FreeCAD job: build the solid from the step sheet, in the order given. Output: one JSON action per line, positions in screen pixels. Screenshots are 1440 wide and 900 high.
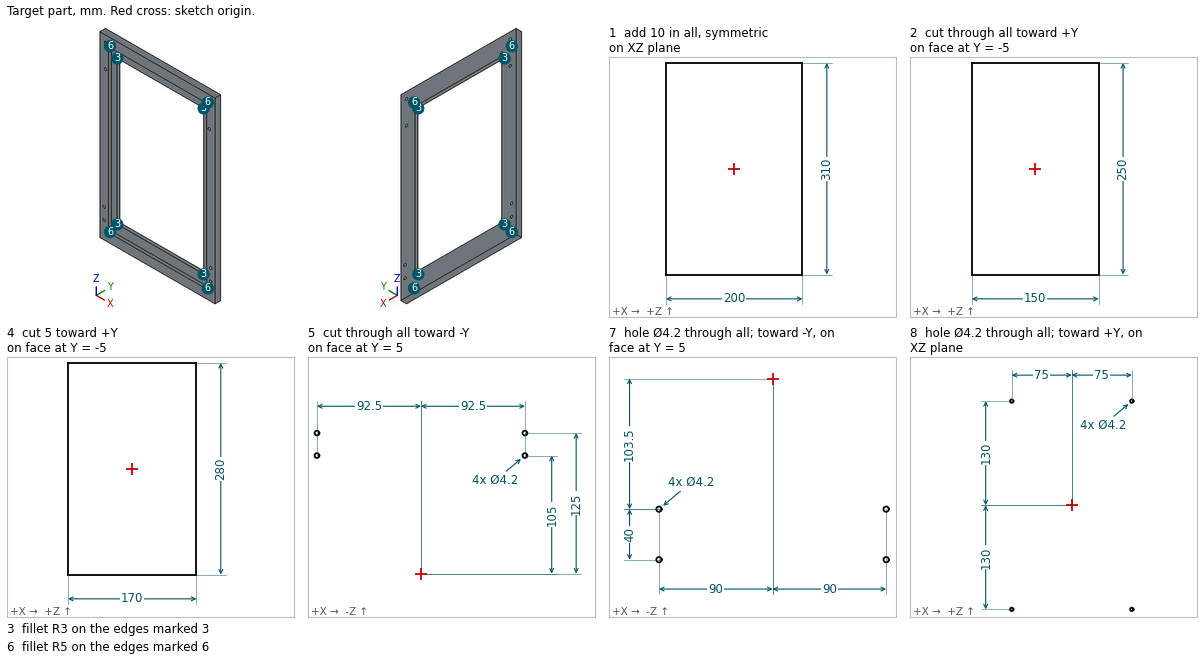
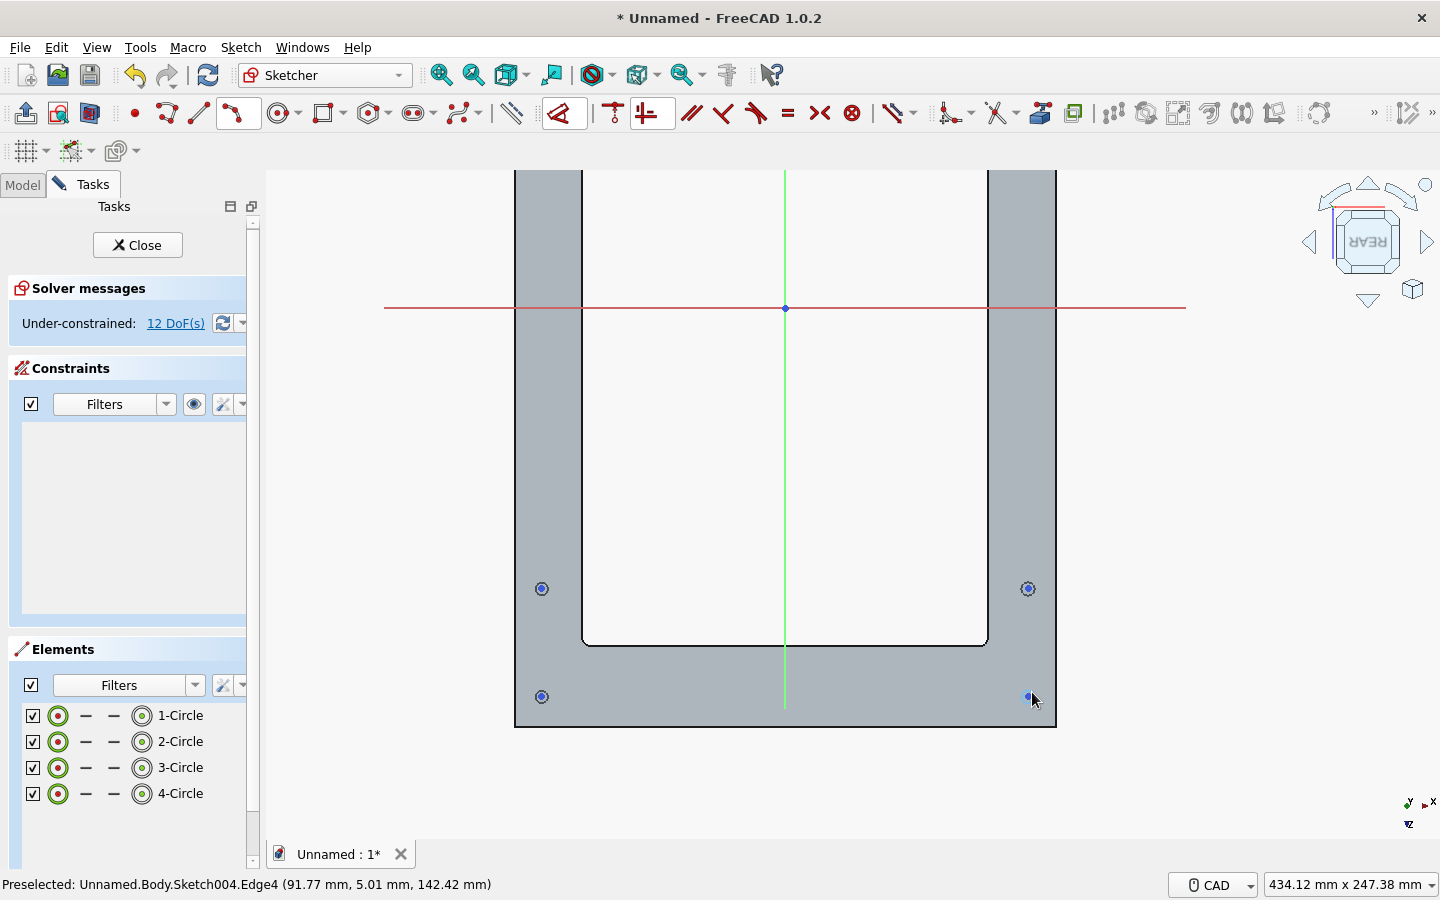
{"action": "scroll", "coordinate": [546, 585], "scroll_direction": "up", "scroll_amount": 4}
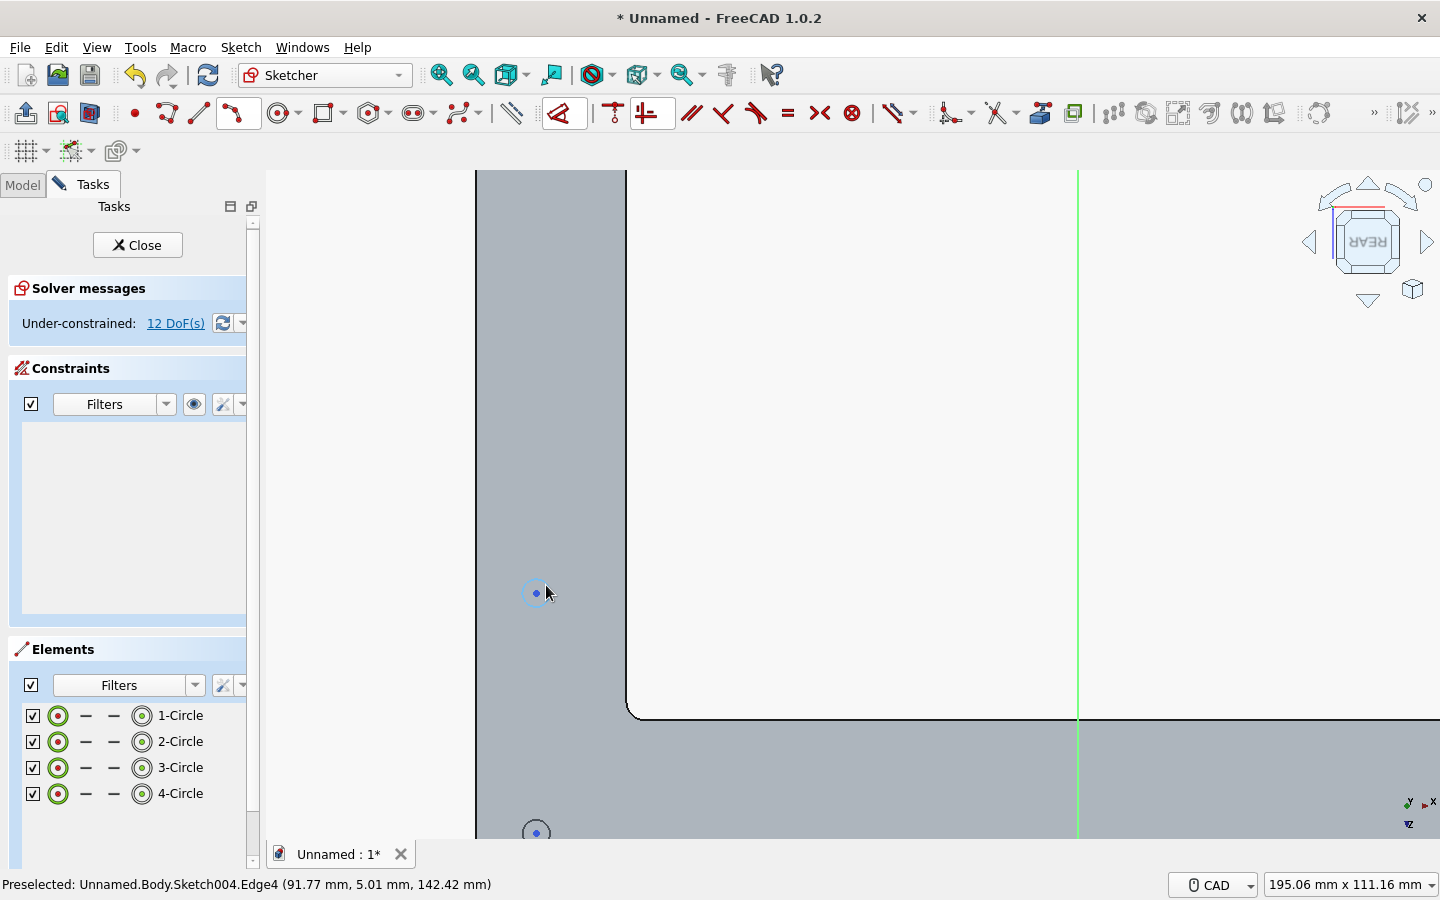
{"action": "left_click", "coordinate": [546, 583]}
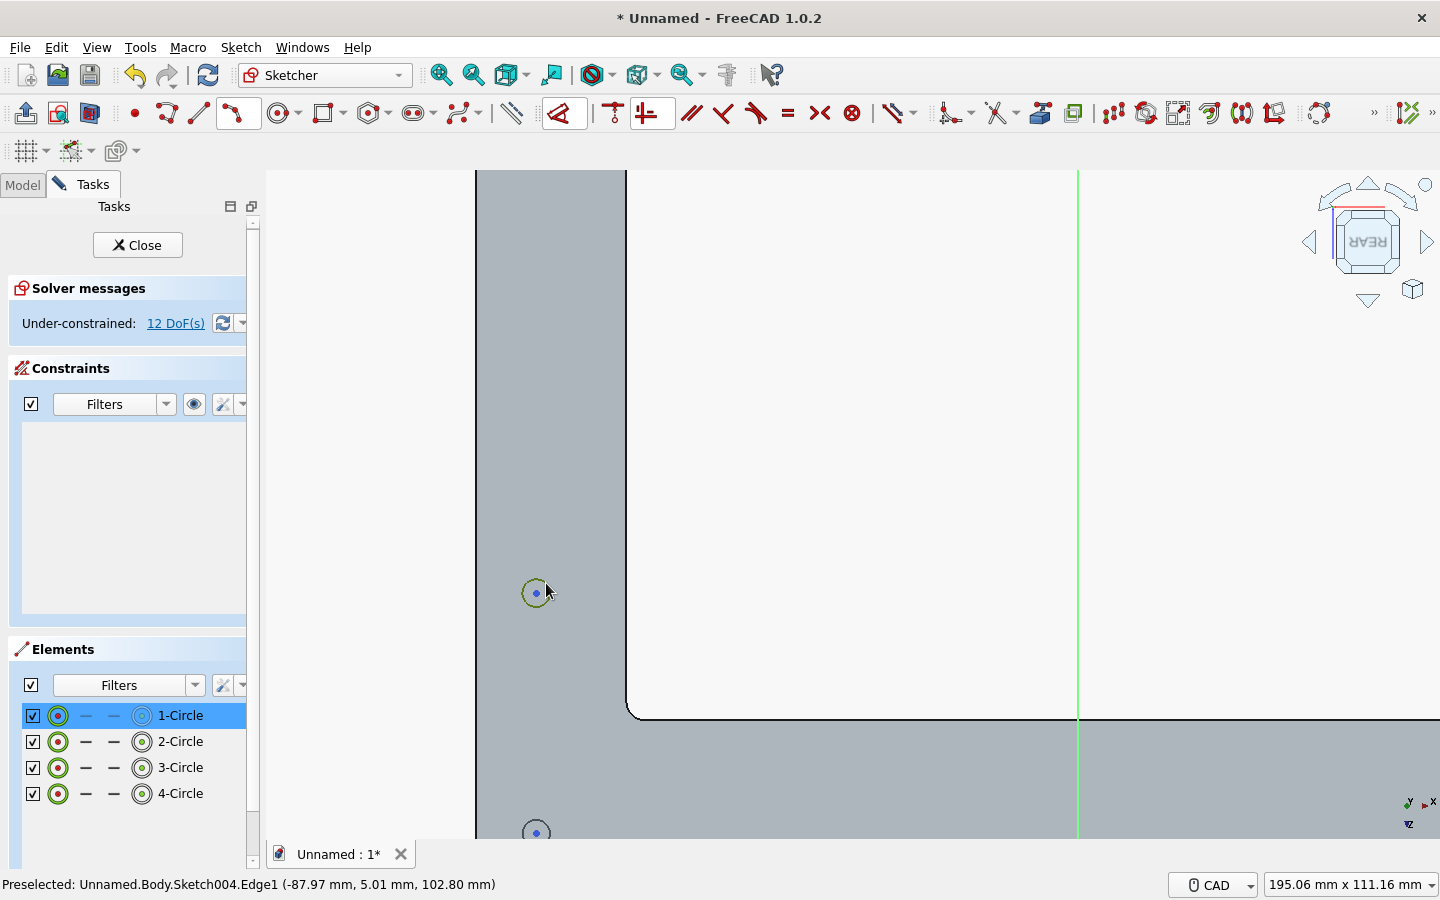
{"action": "scroll", "coordinate": [545, 585], "scroll_direction": "down", "scroll_amount": 4}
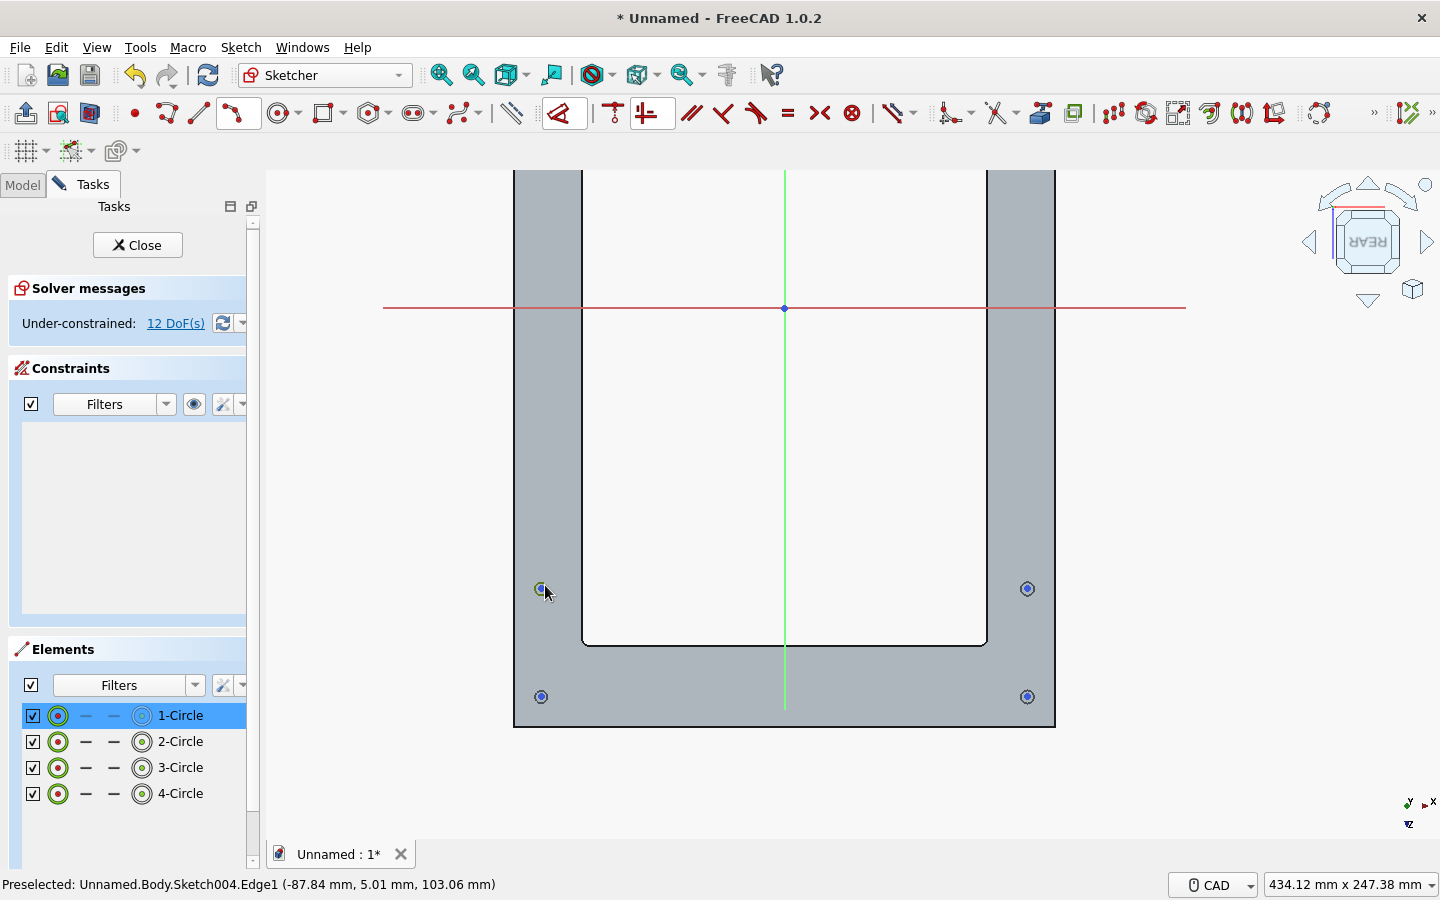
{"action": "scroll", "coordinate": [546, 693], "scroll_direction": "up", "scroll_amount": 5}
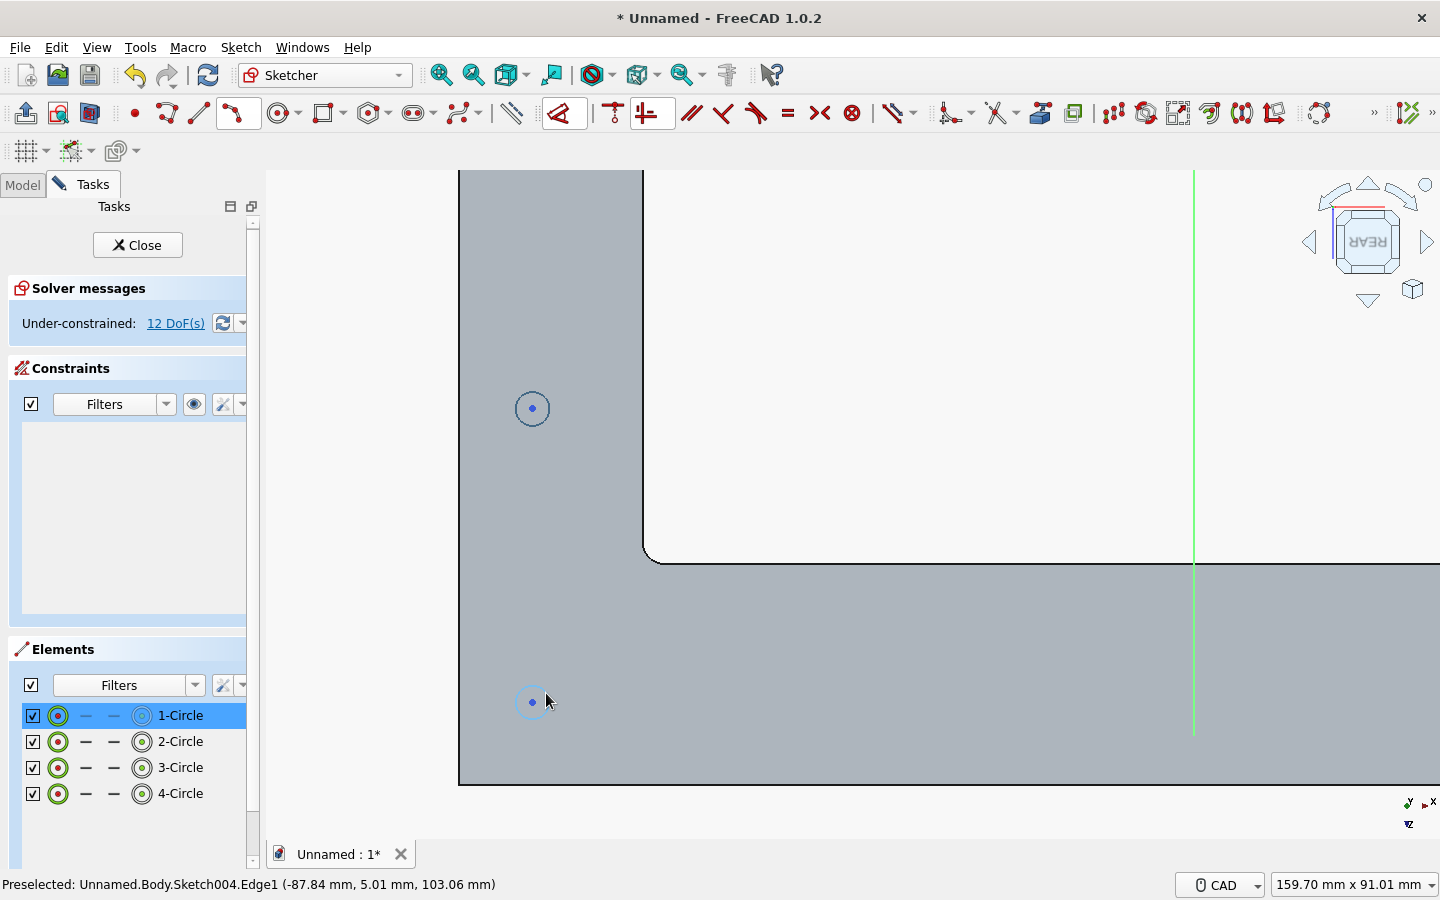
{"action": "left_click", "coordinate": [544, 691]}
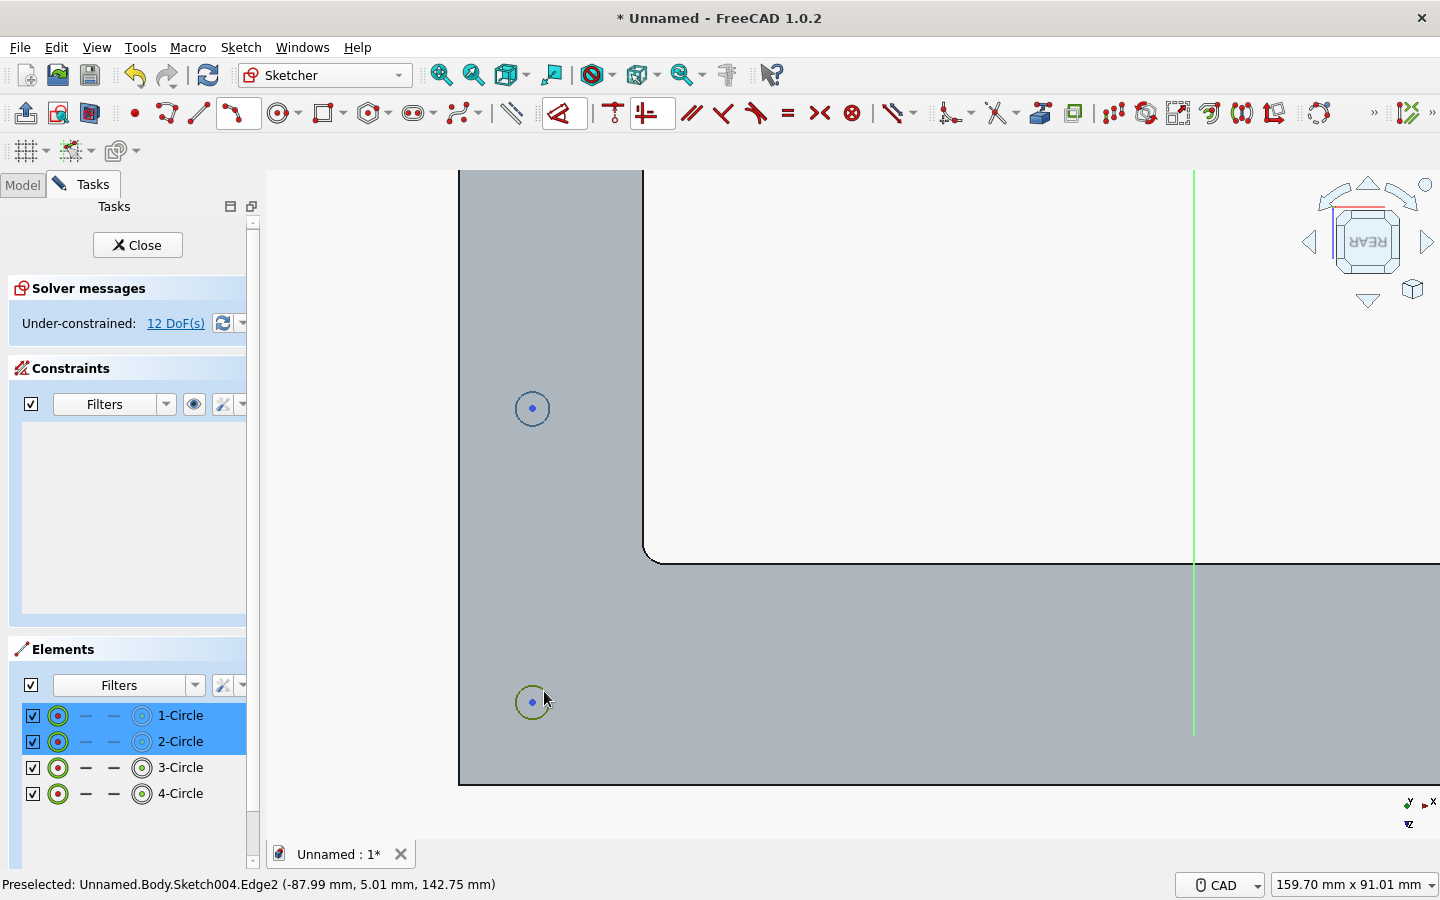
{"action": "scroll", "coordinate": [546, 693], "scroll_direction": "down", "scroll_amount": 5}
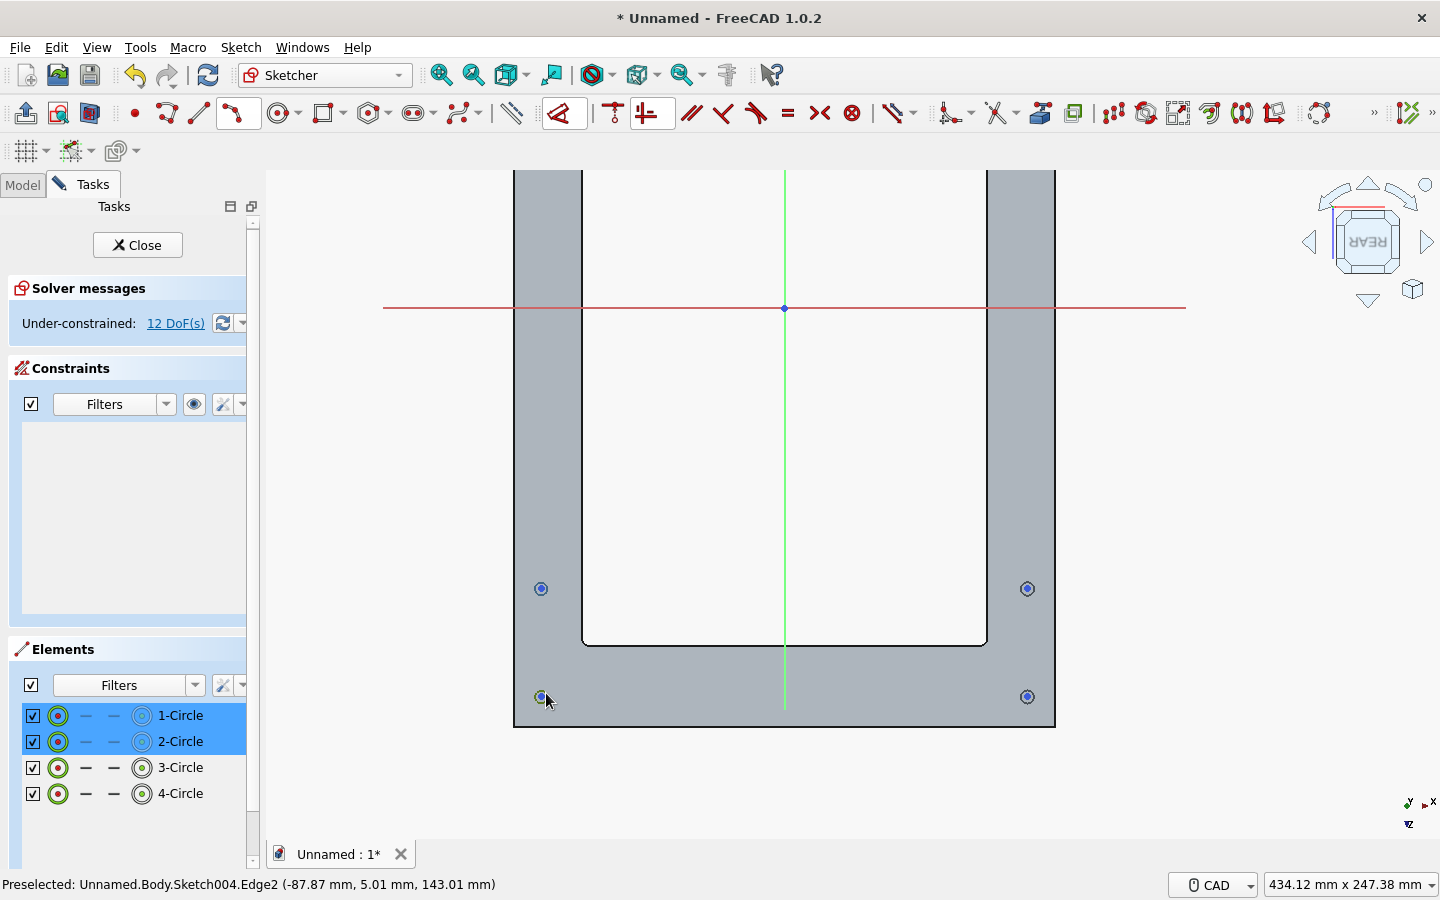
{"action": "scroll", "coordinate": [1032, 584], "scroll_direction": "up", "scroll_amount": 4}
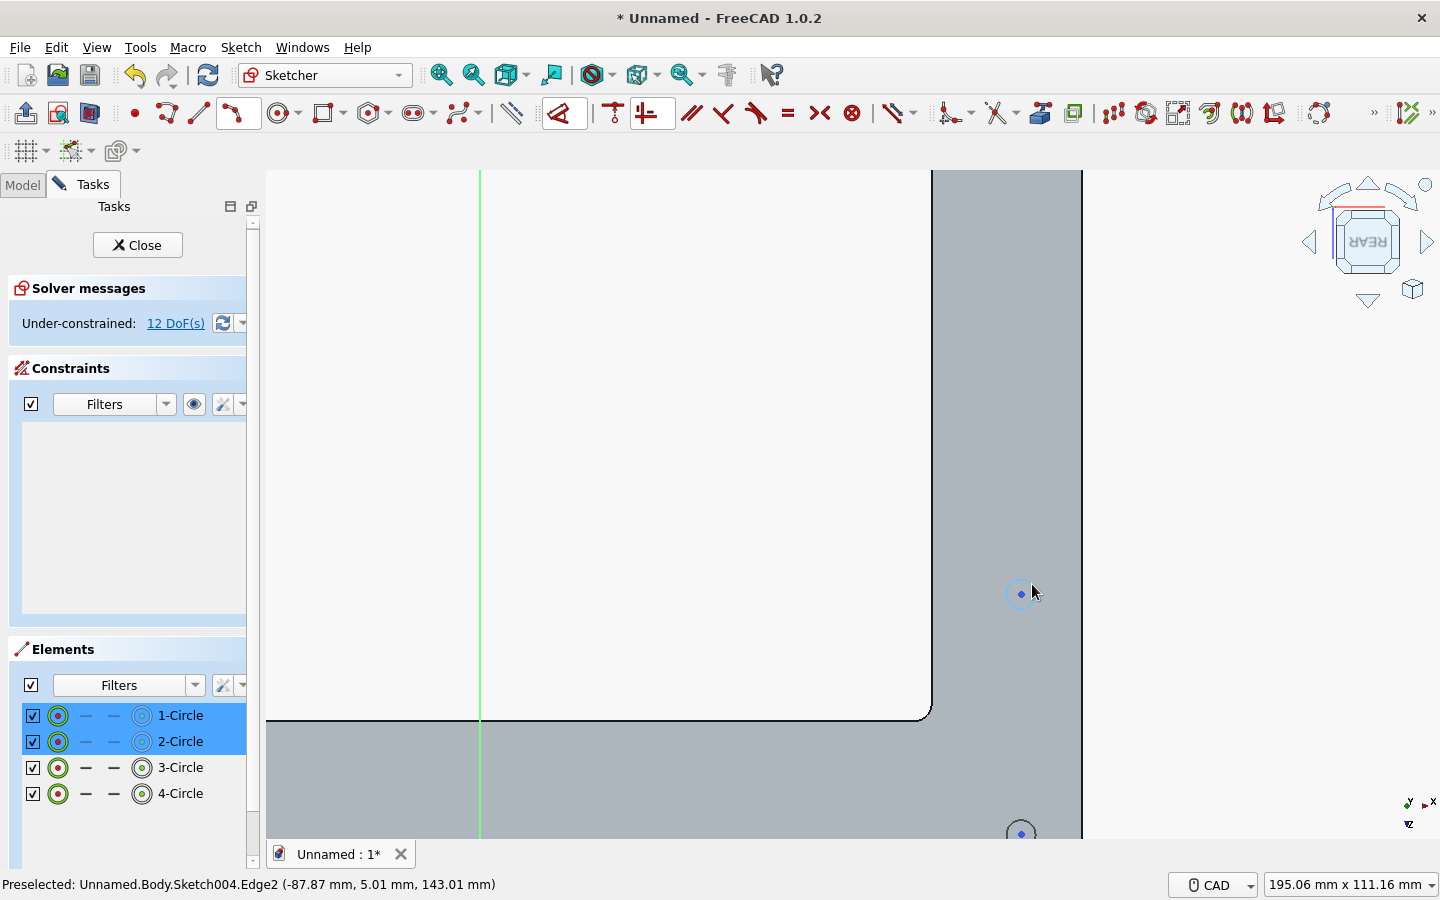
{"action": "left_click", "coordinate": [1031, 584]}